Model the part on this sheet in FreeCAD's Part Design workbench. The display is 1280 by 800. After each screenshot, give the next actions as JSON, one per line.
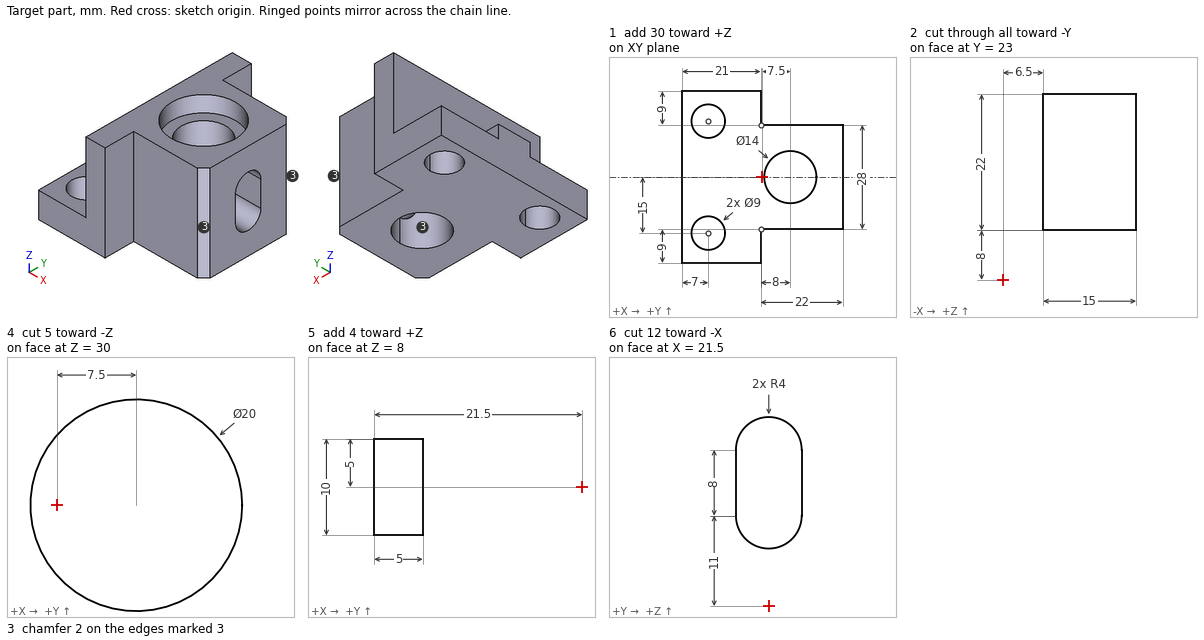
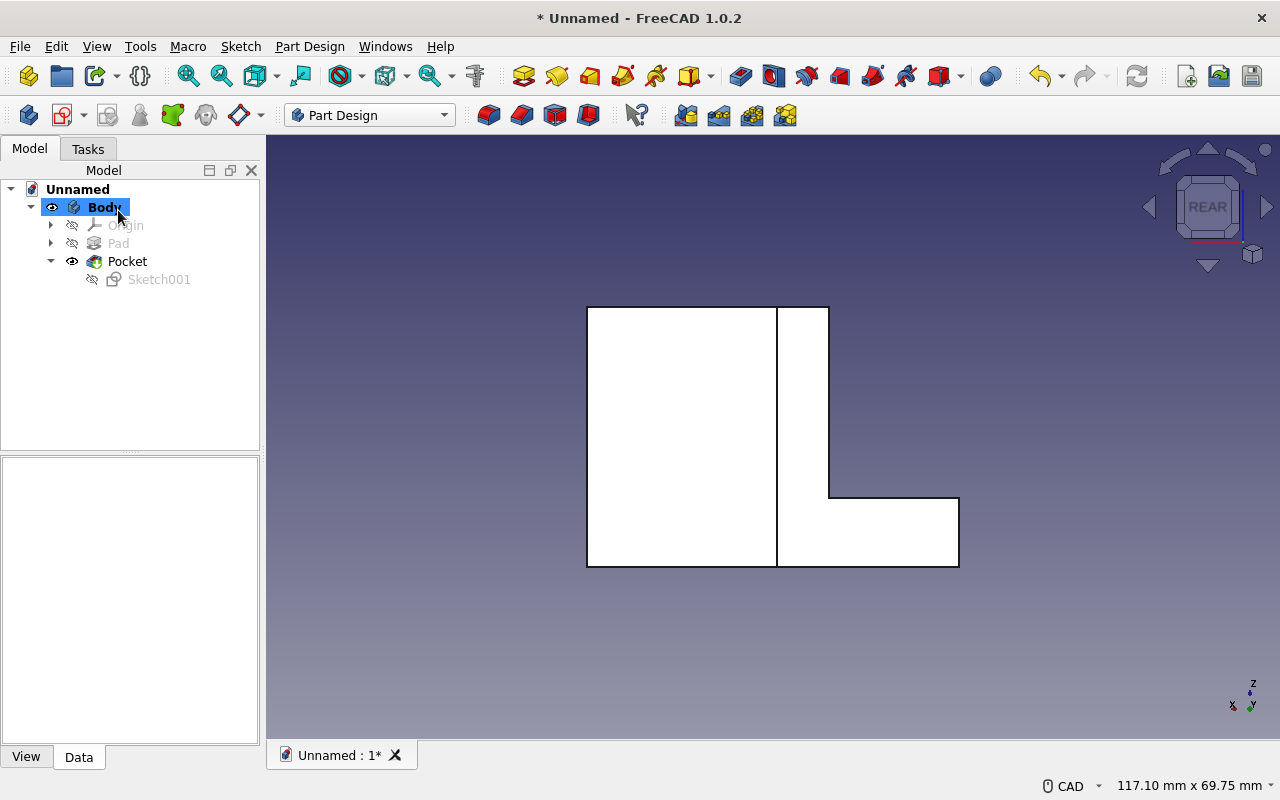
{"action": "key", "text": "0"}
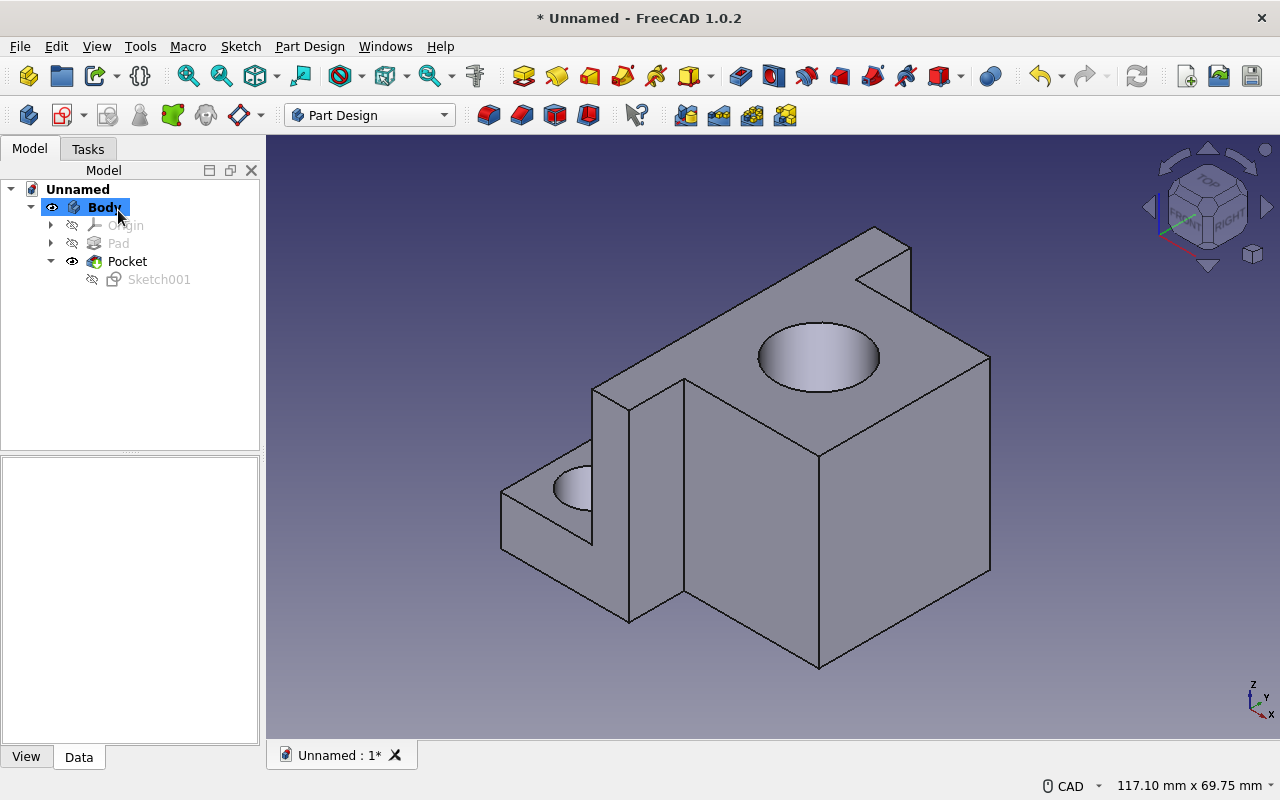
{"action": "left_click", "coordinate": [819, 562]}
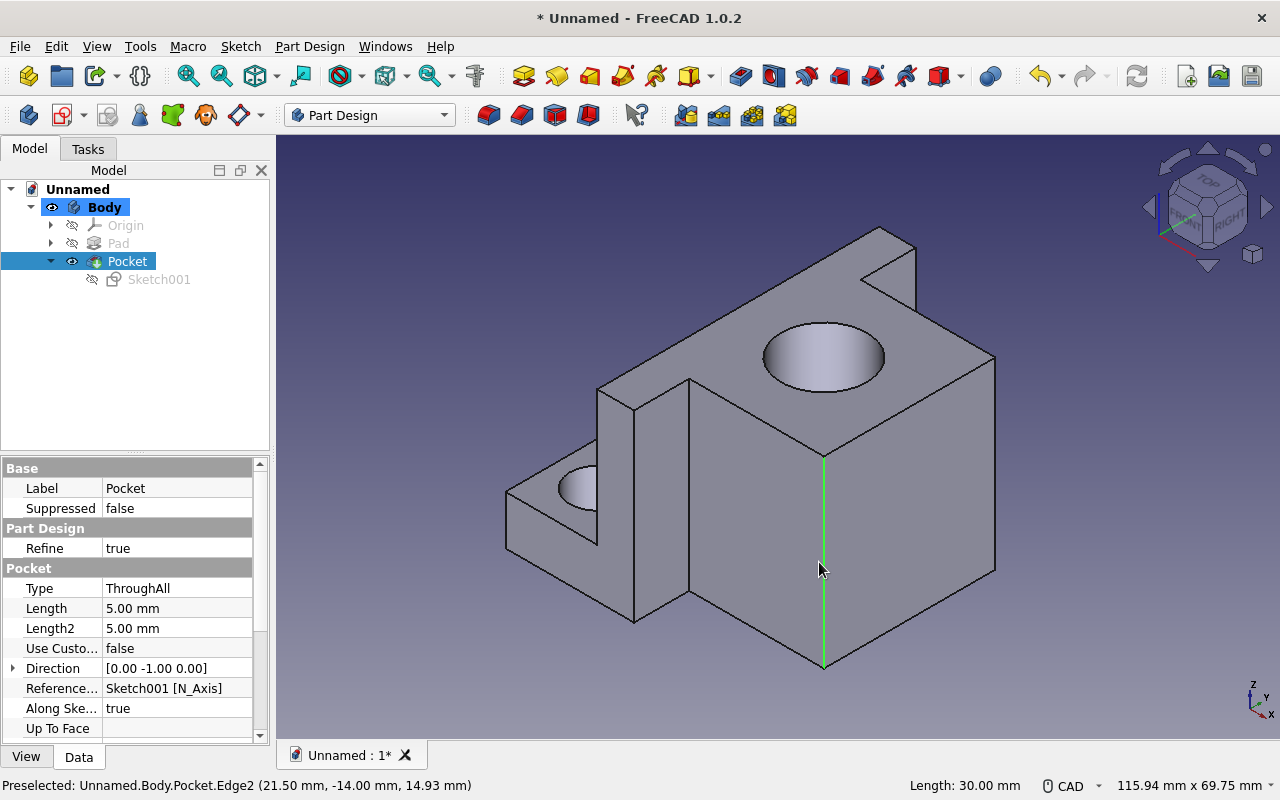
{"action": "key", "text": "2"}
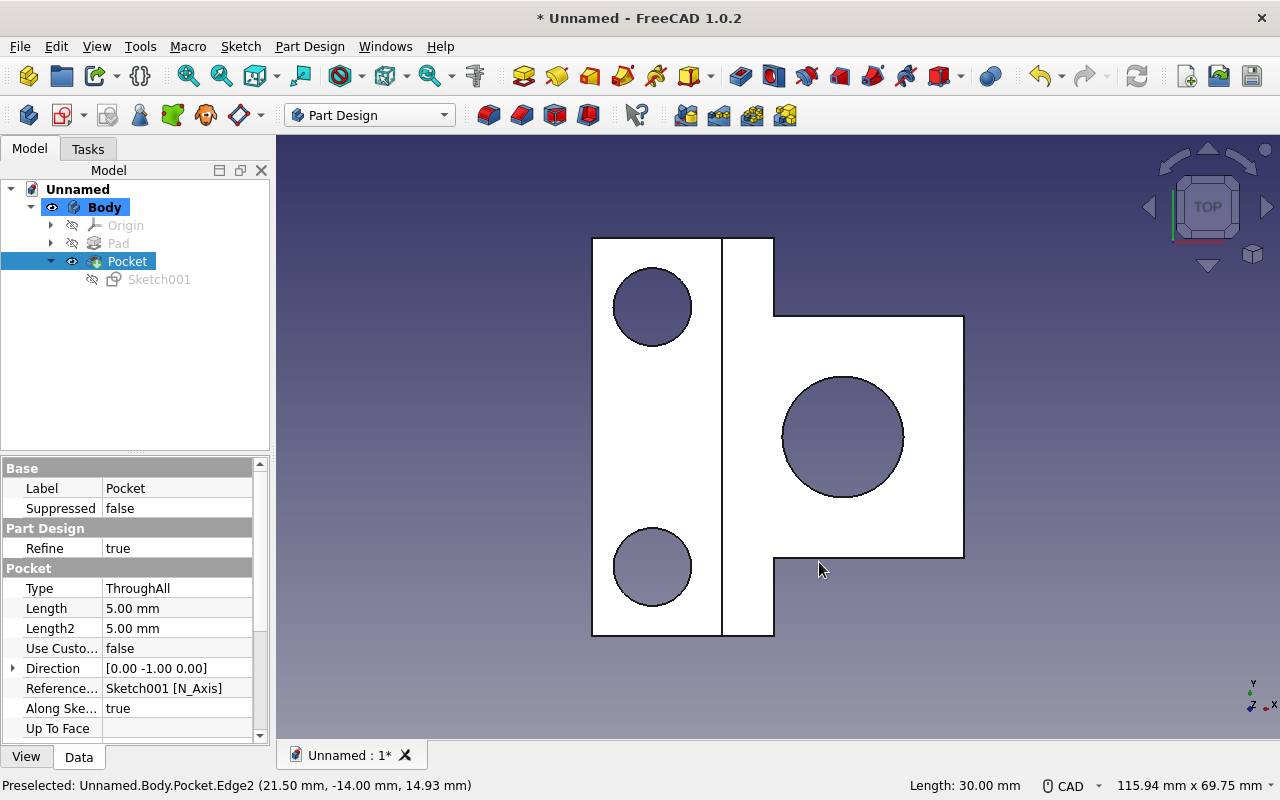
{"action": "key", "text": "1"}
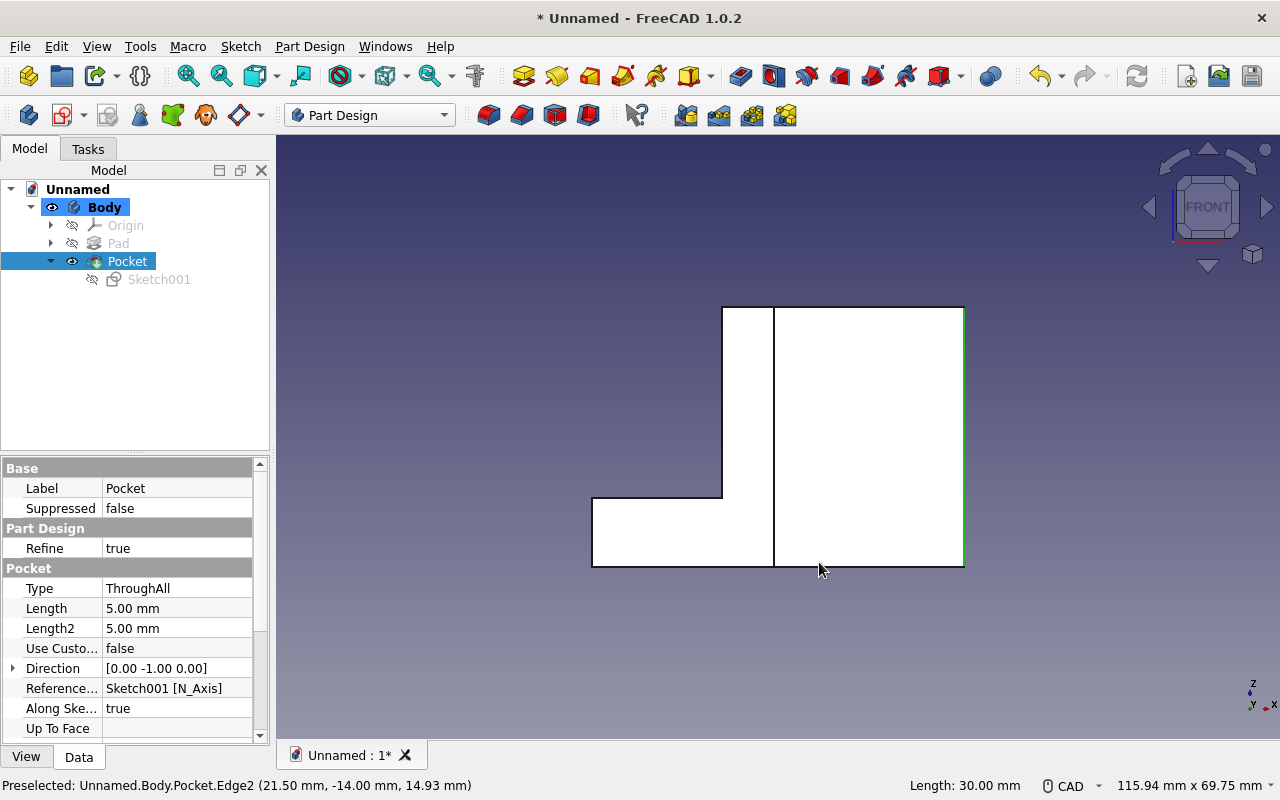
{"action": "left_click", "coordinate": [189, 76]}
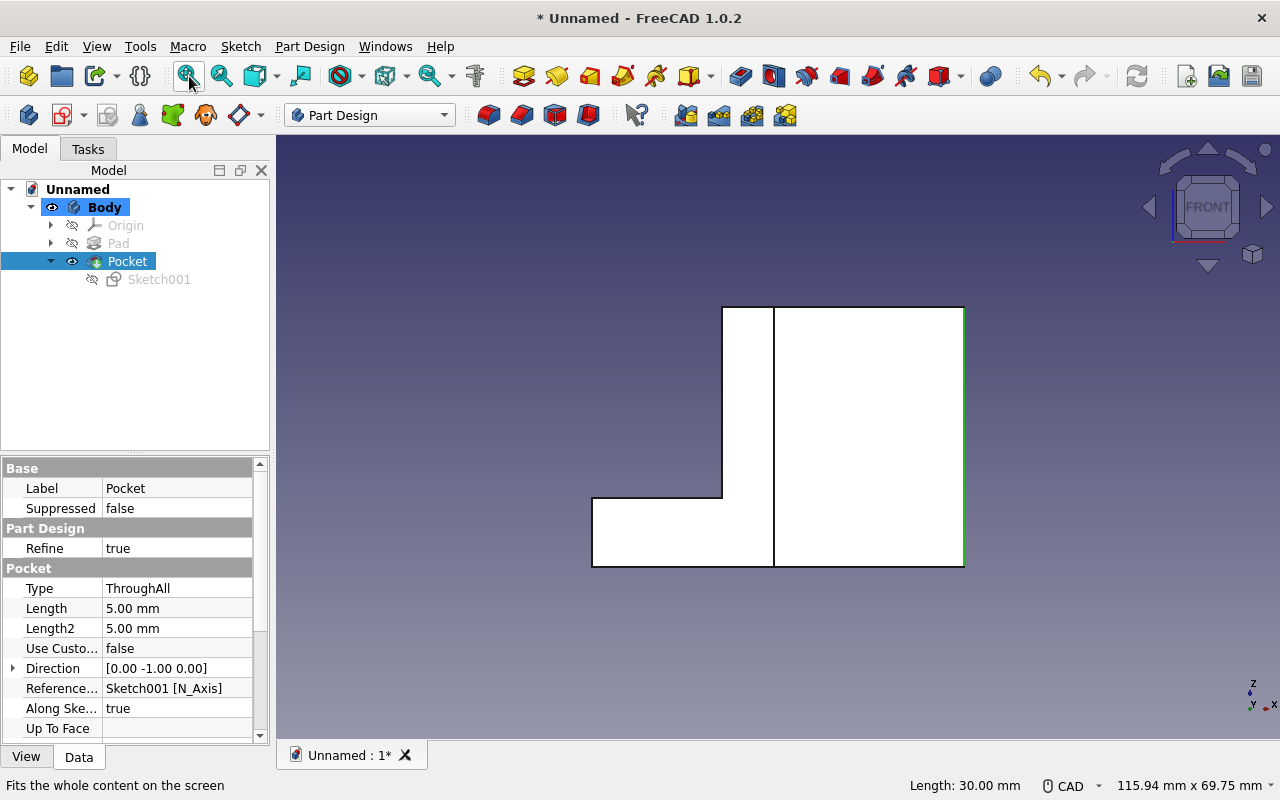
{"action": "key", "text": "3"}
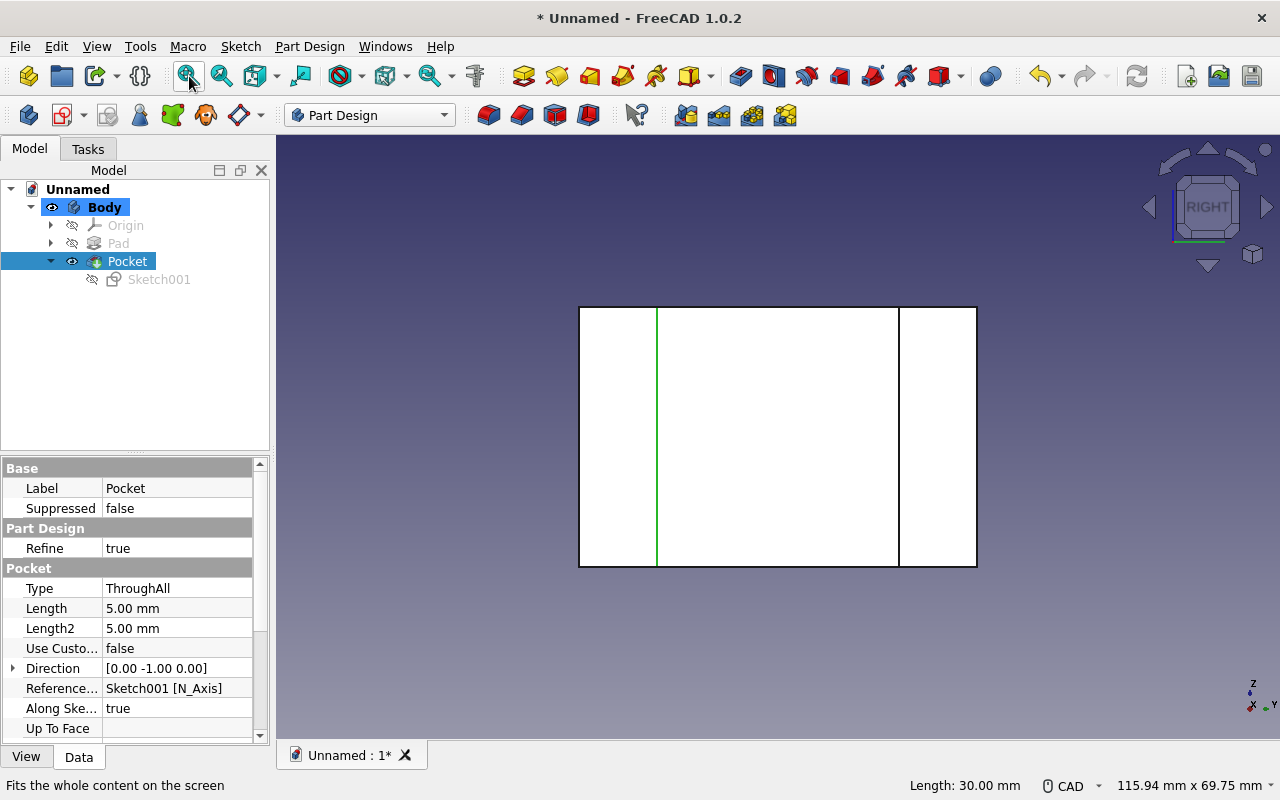
{"action": "key", "text": "v f"}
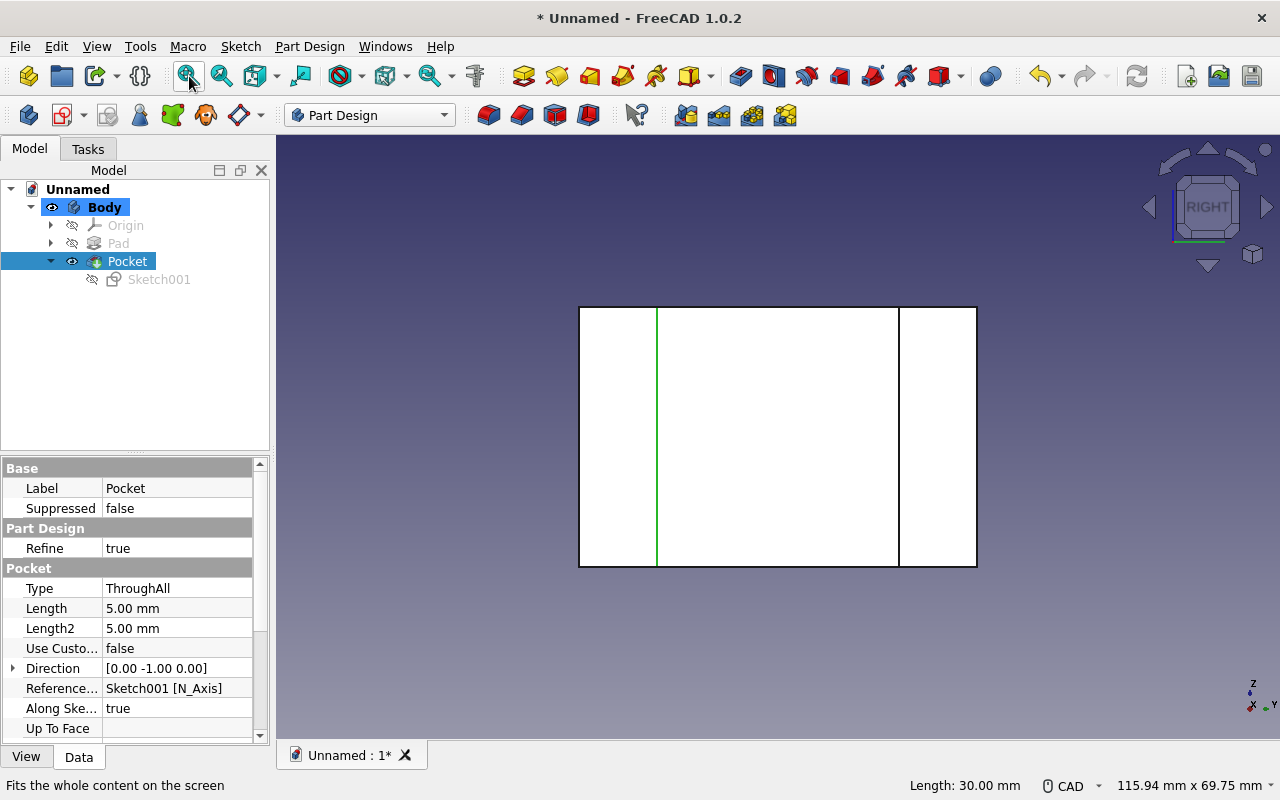
{"action": "left_click", "coordinate": [899, 436], "text": "ctrl"}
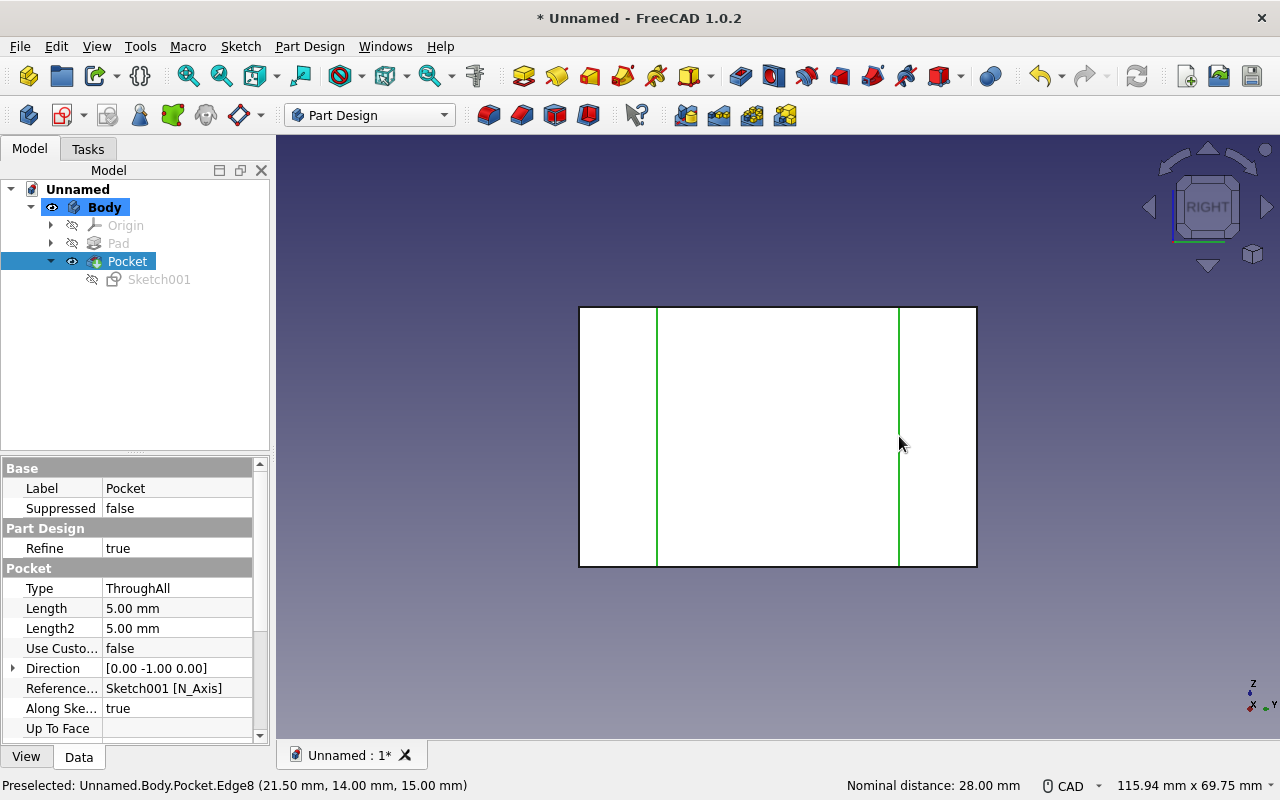
{"action": "left_click", "coordinate": [522, 116]}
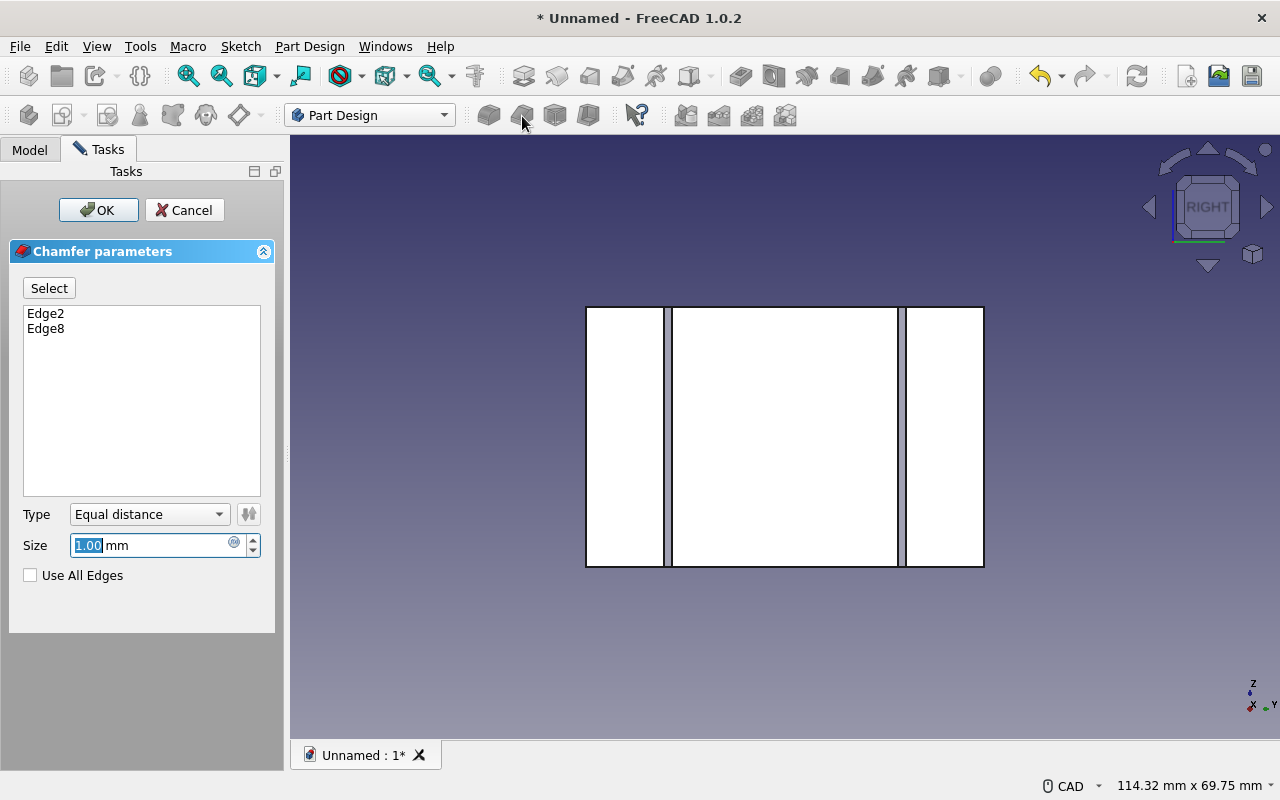
{"action": "type", "text": "2"}
{"action": "key", "text": "Tab"}